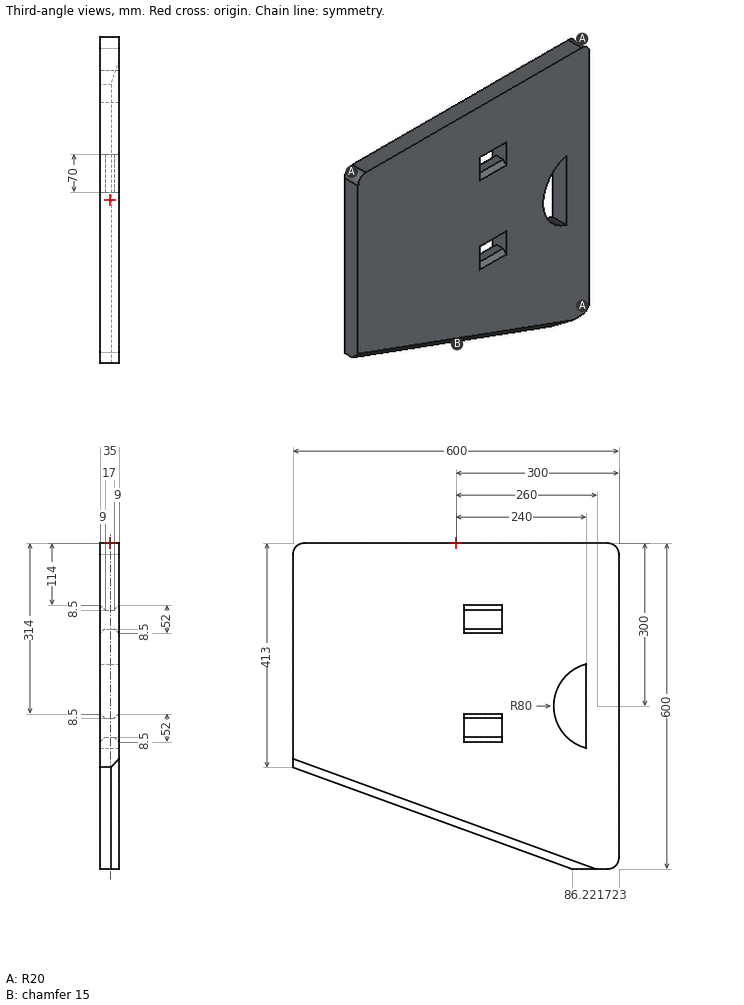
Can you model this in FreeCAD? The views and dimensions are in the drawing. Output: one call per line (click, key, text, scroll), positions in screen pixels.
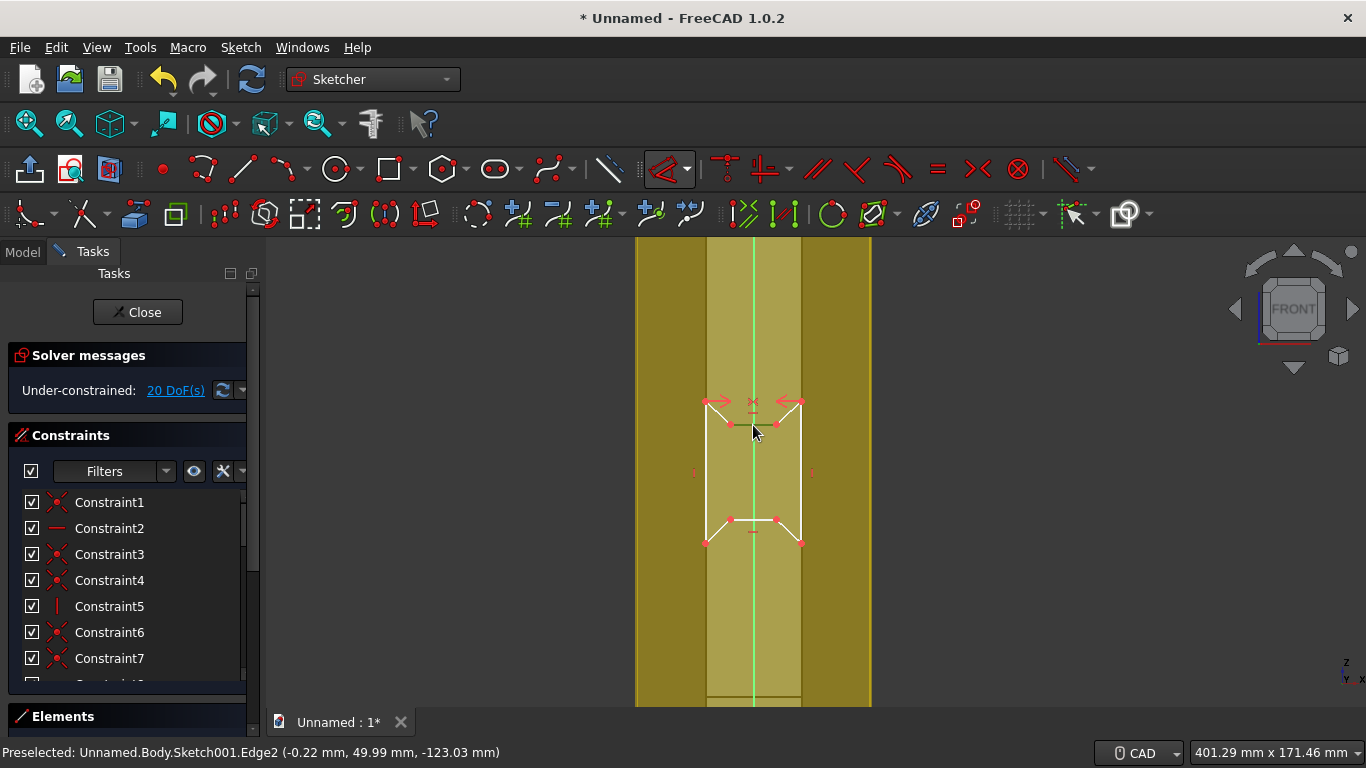
click(690, 170)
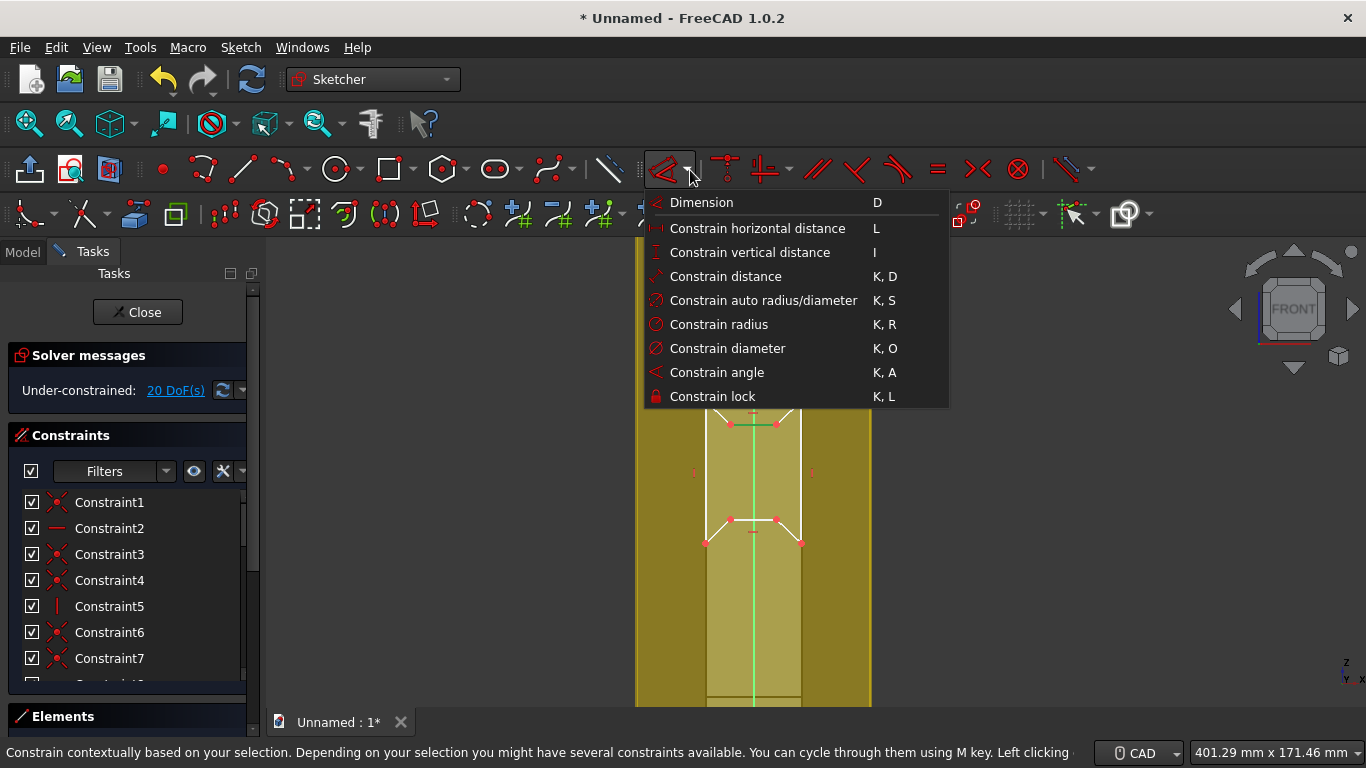
click(797, 228)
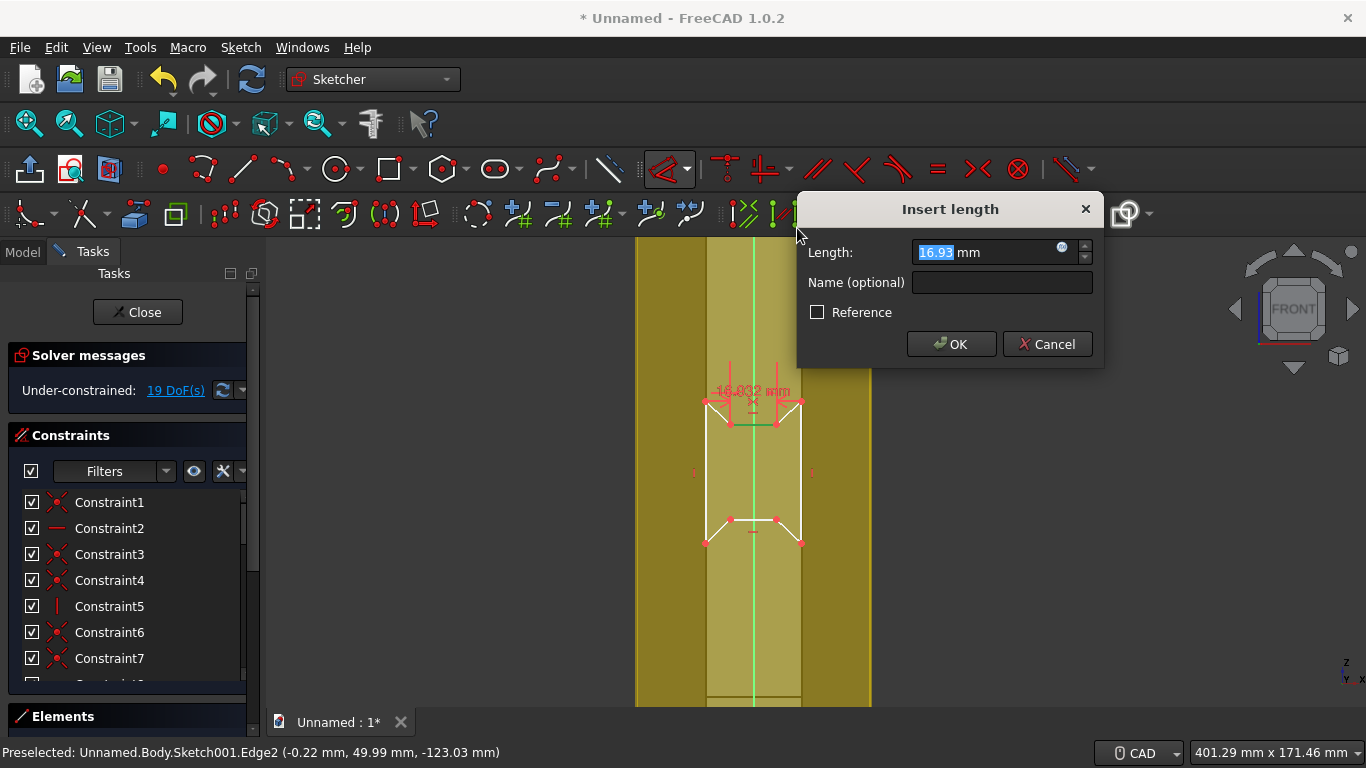
text(17)
key(Return)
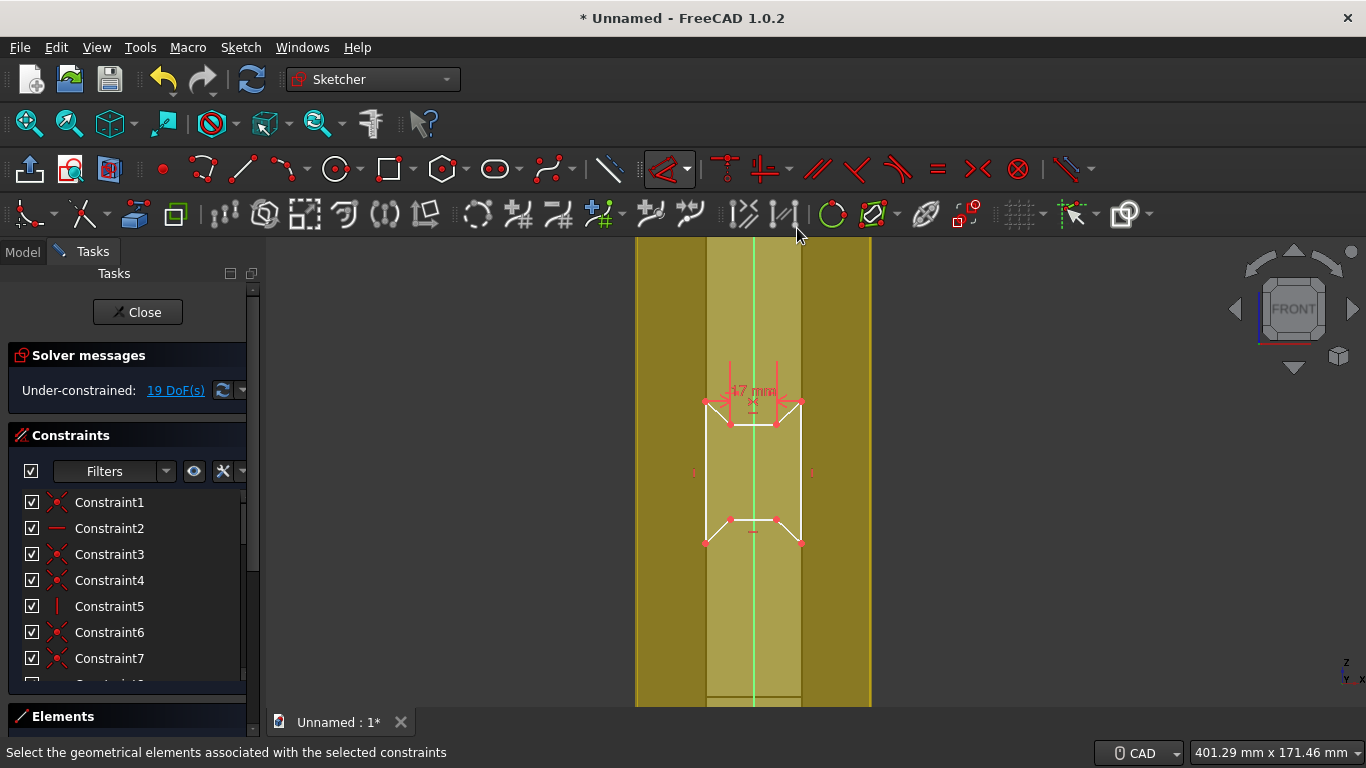
click(801, 444)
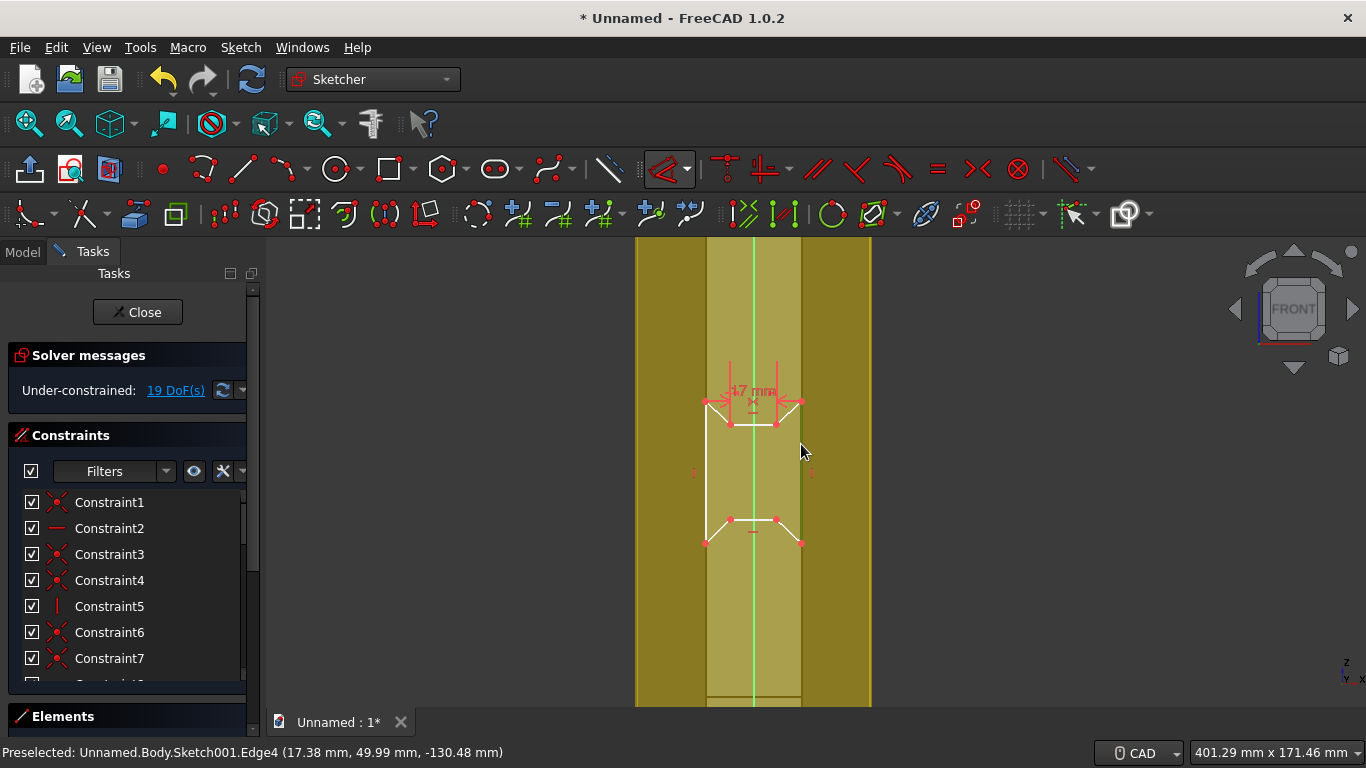
key(i)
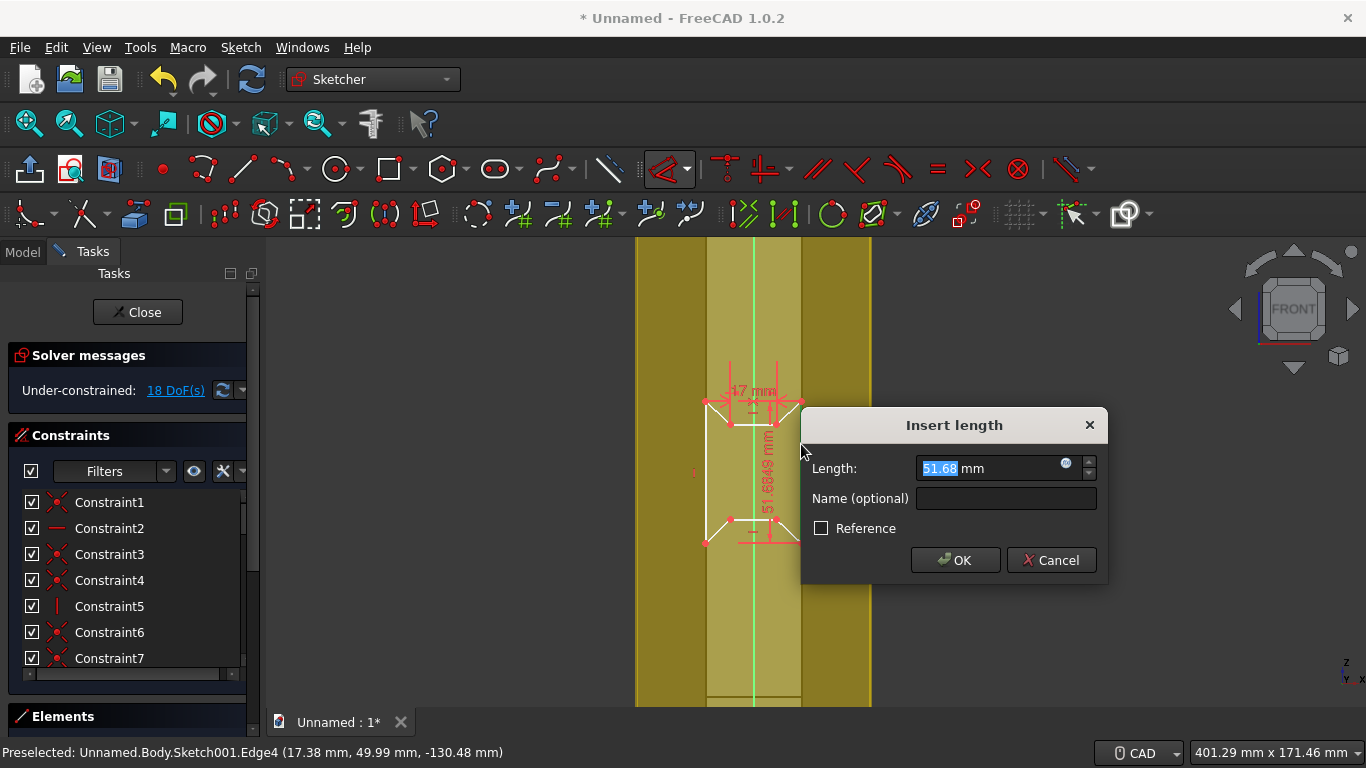
text(52)
key(Return)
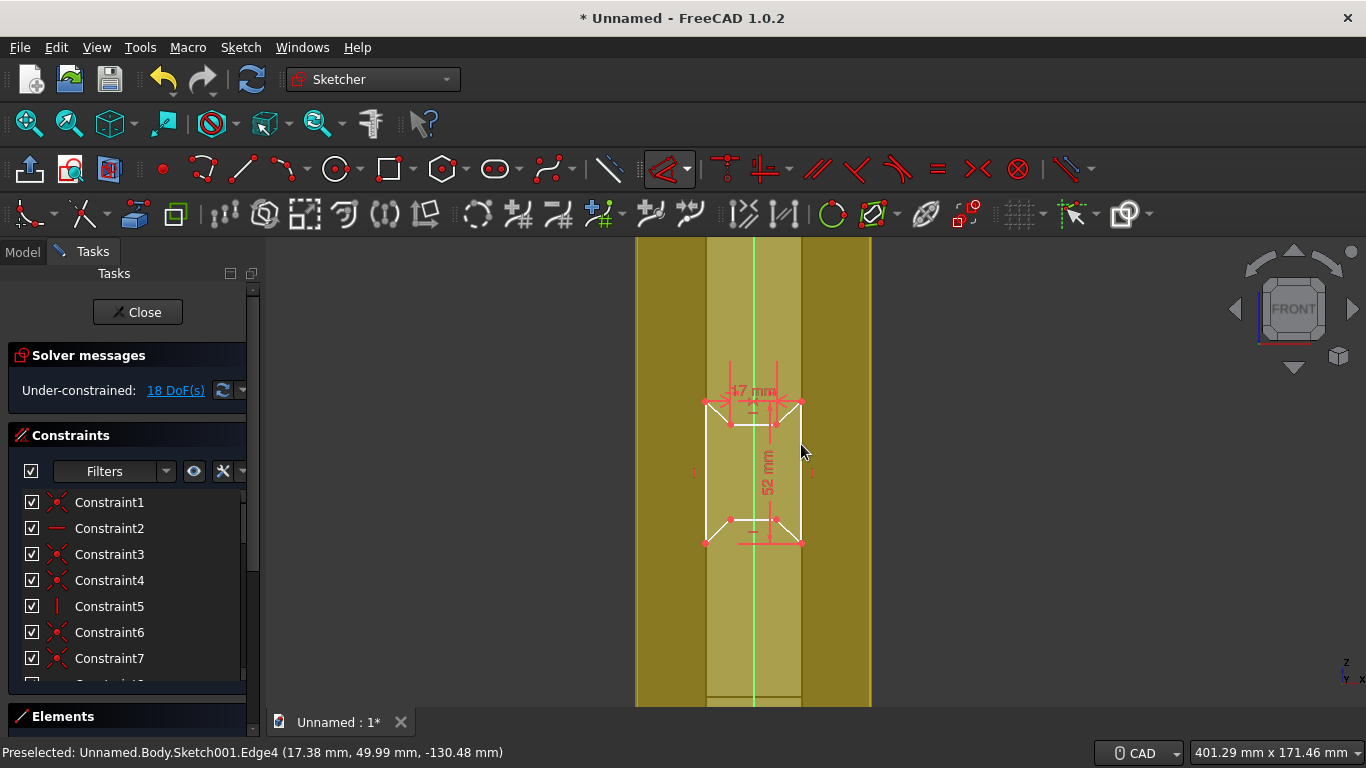
scroll(763, 520, up, 3)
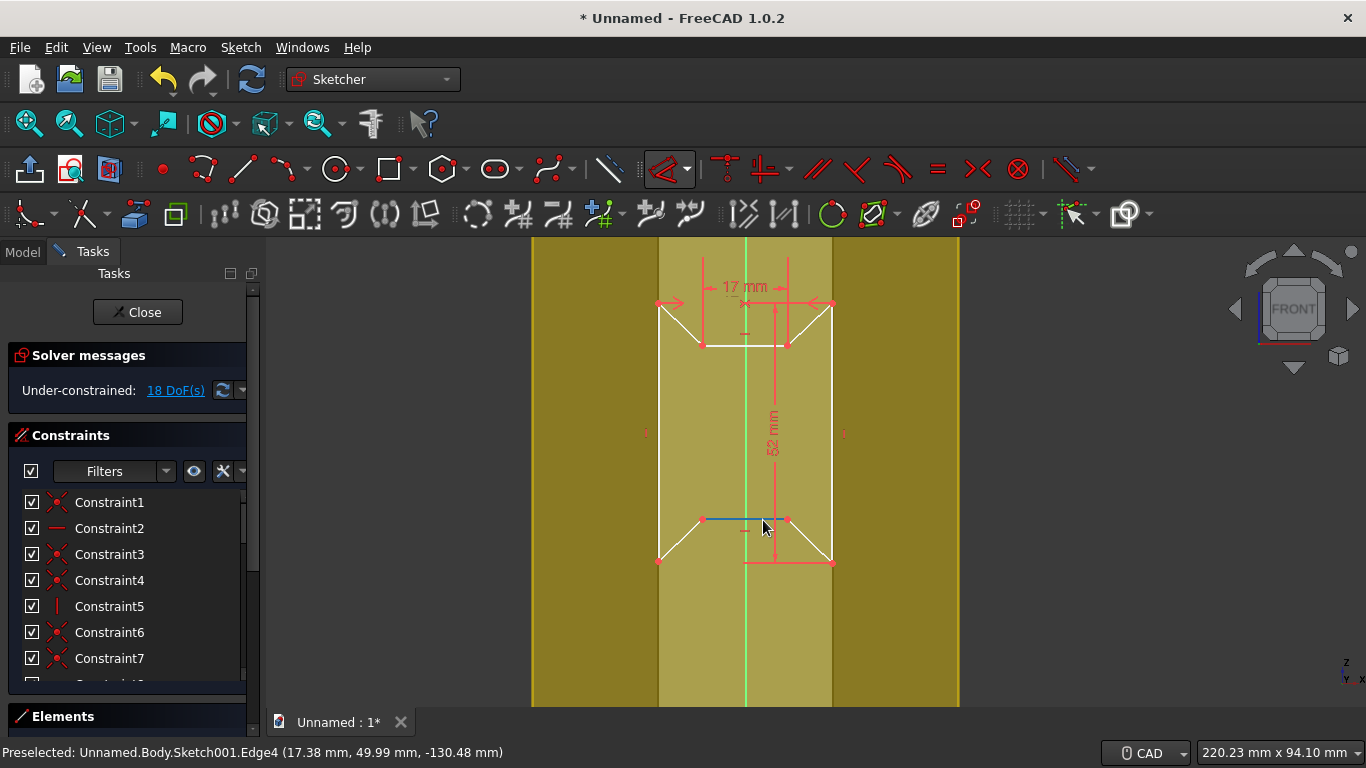
click(762, 519)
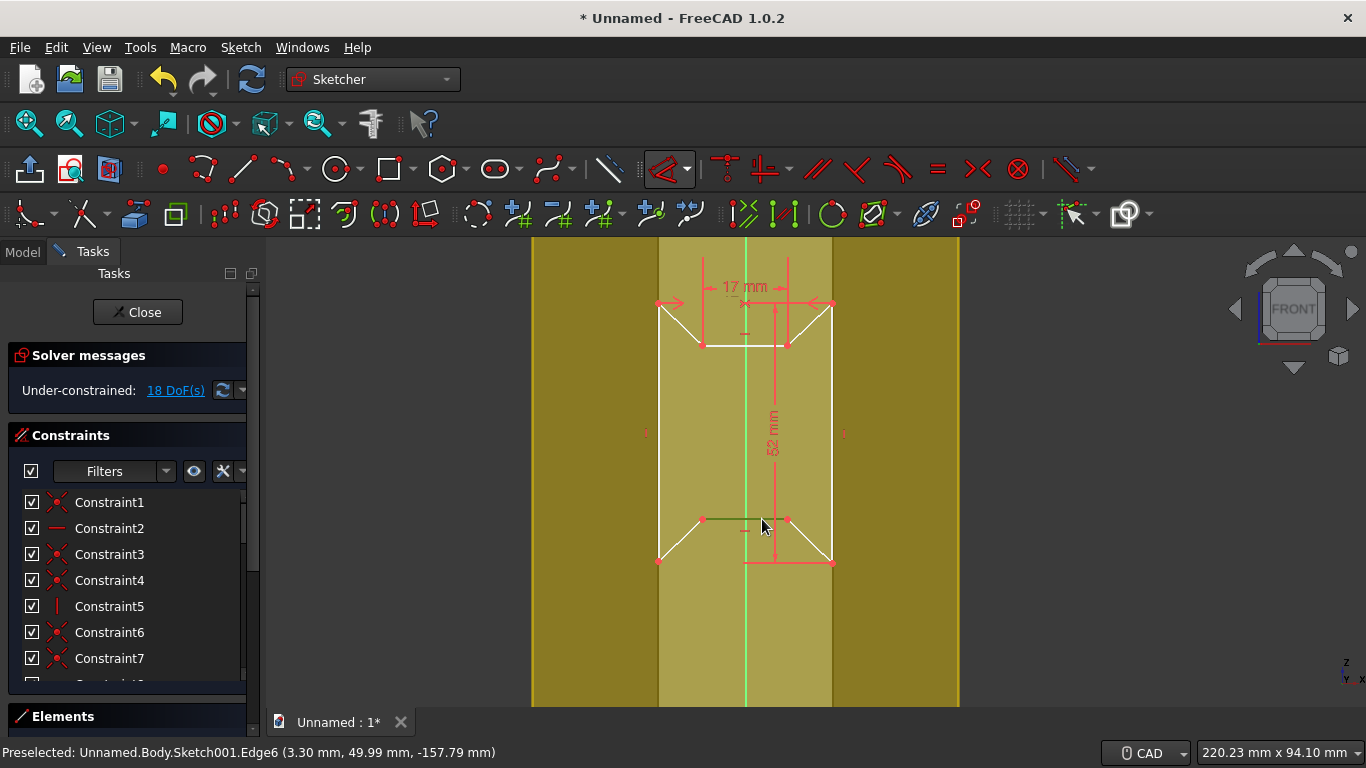
click(690, 170)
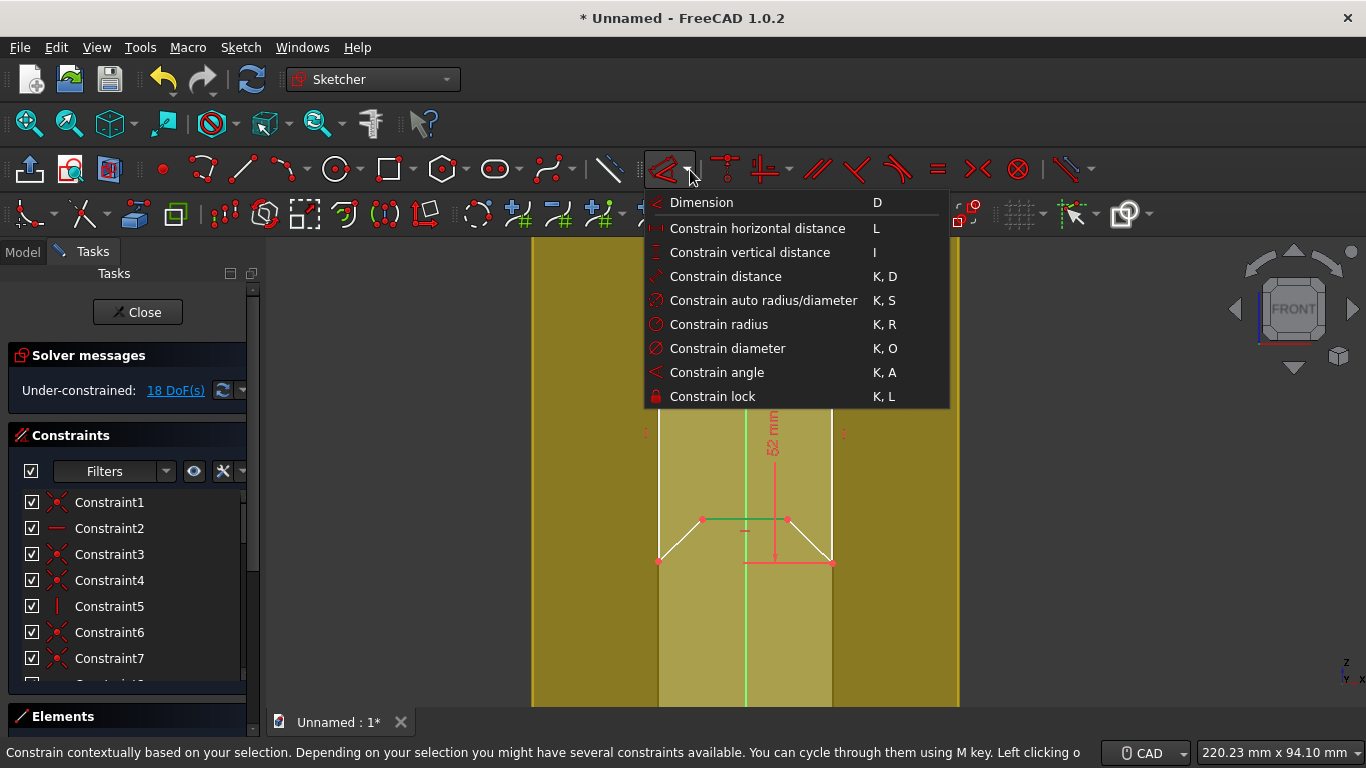
click(797, 228)